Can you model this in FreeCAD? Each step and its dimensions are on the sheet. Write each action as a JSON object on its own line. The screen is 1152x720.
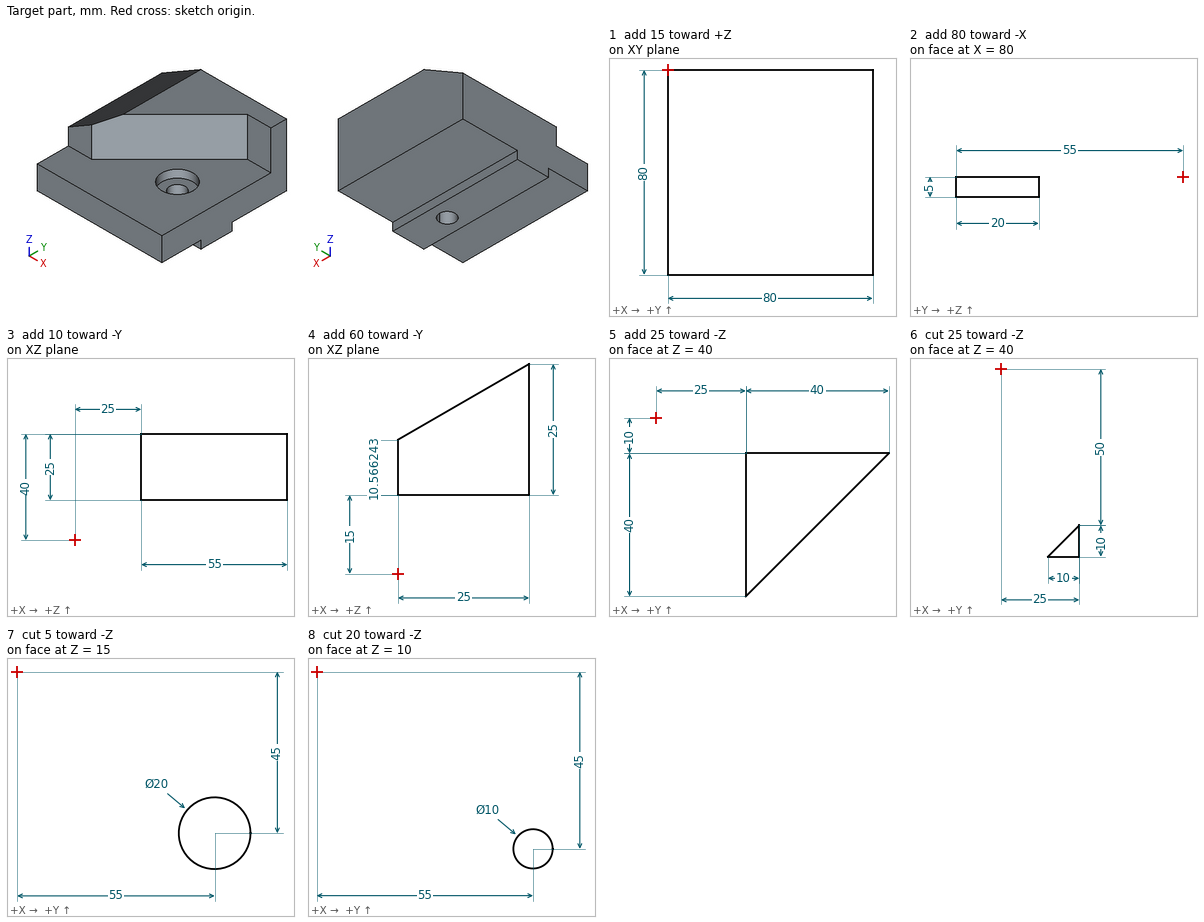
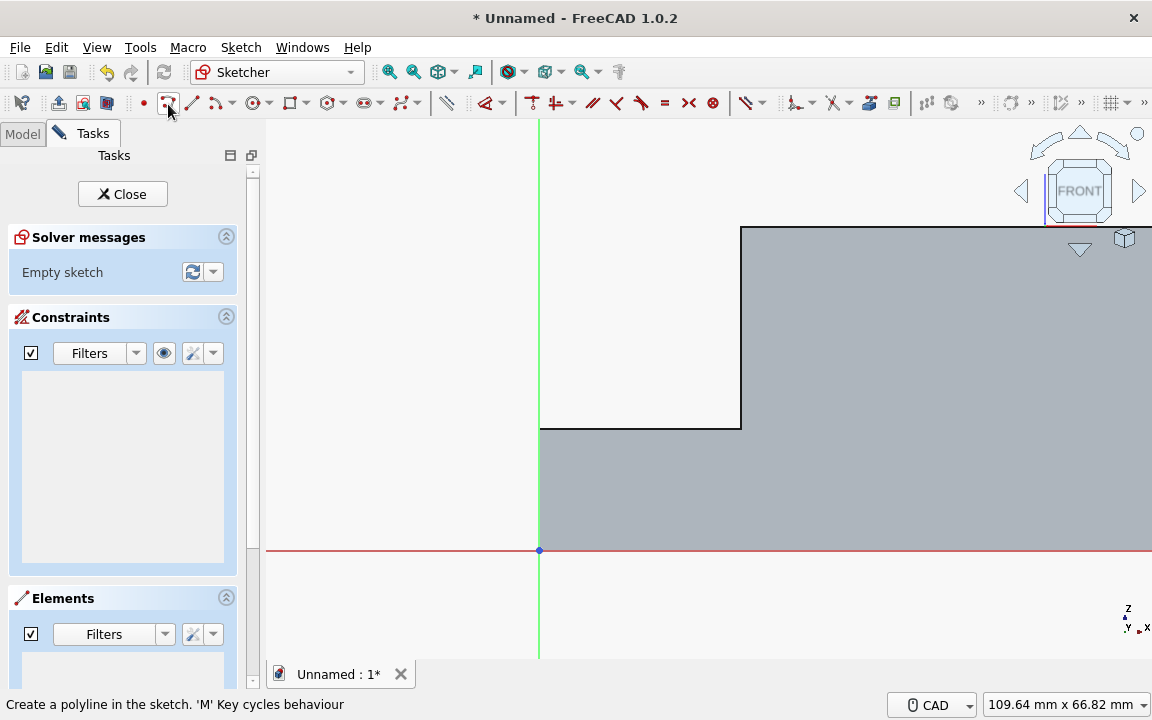
{"action": "left_click", "coordinate": [539, 429]}
{"action": "left_click", "coordinate": [548, 344]}
{"action": "left_click", "coordinate": [741, 227]}
{"action": "left_click", "coordinate": [741, 429]}
{"action": "left_click", "coordinate": [539, 430]}
{"action": "key", "text": "Escape"}
{"action": "key", "text": "Escape"}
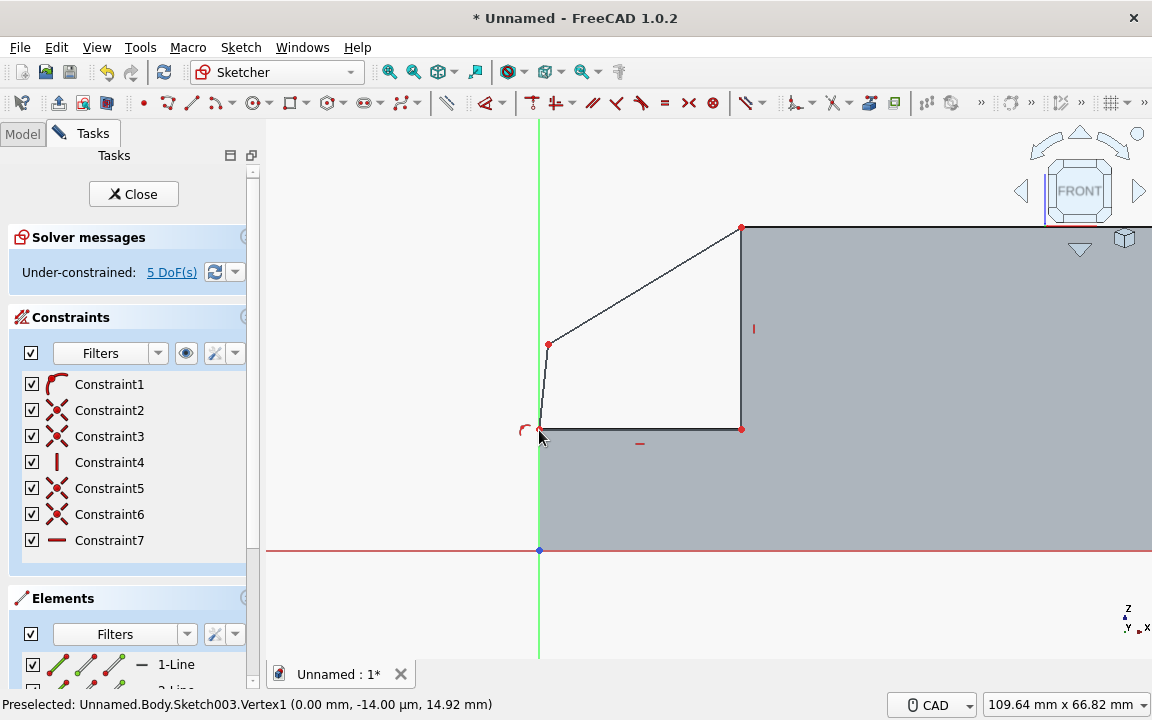
{"action": "left_click", "coordinate": [542, 404]}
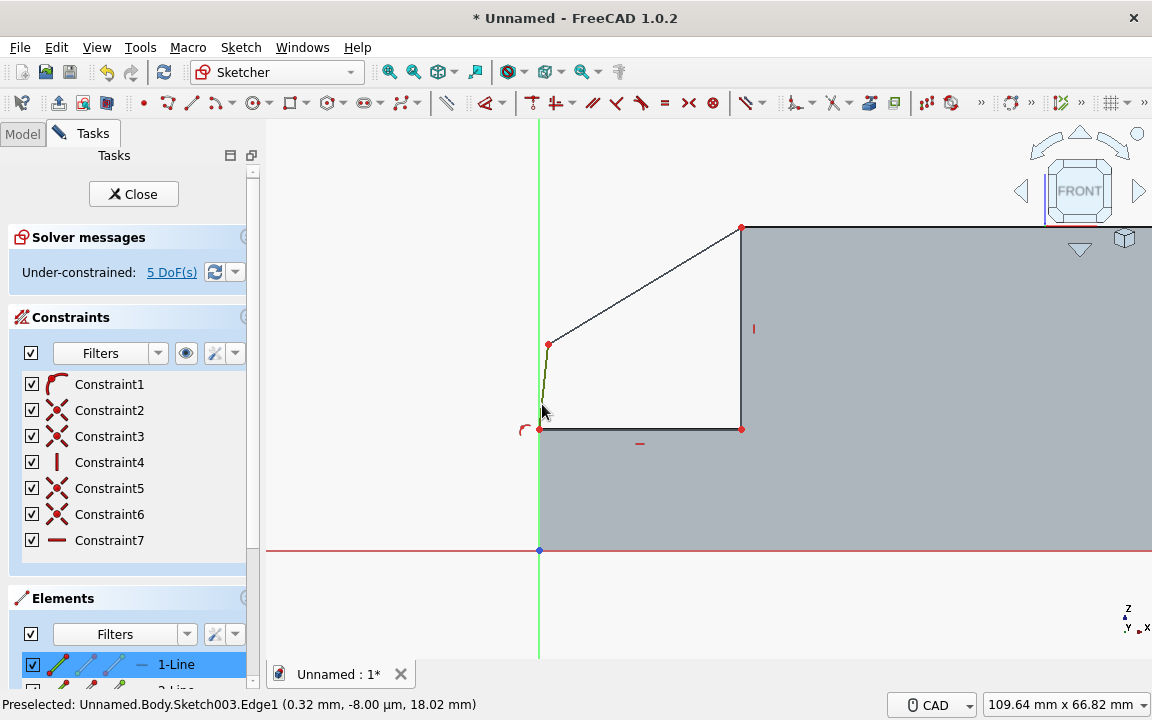
{"action": "left_click", "coordinate": [574, 104]}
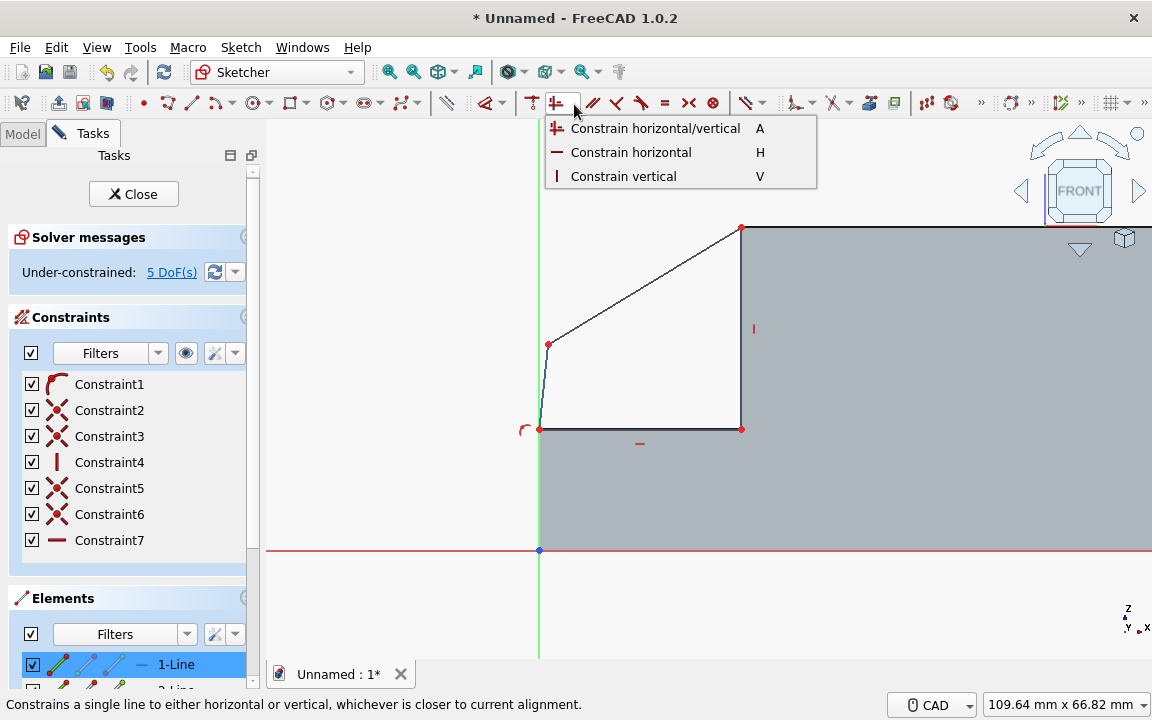
{"action": "left_click", "coordinate": [681, 176]}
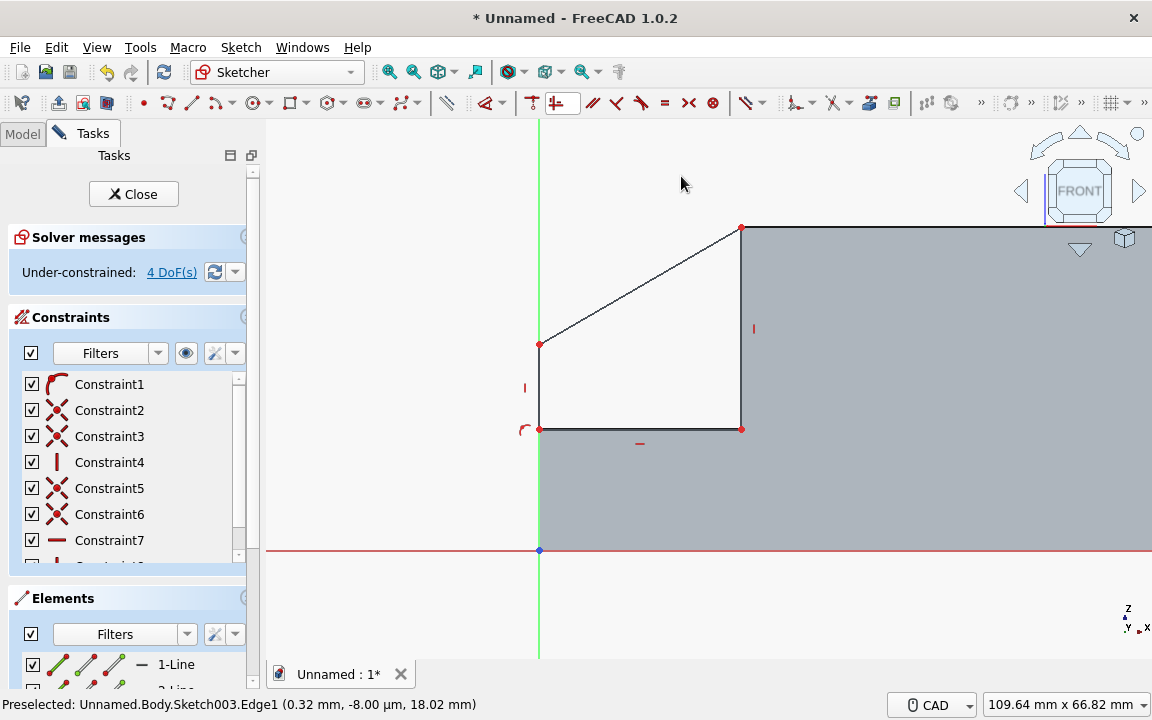
{"action": "left_click", "coordinate": [486, 104]}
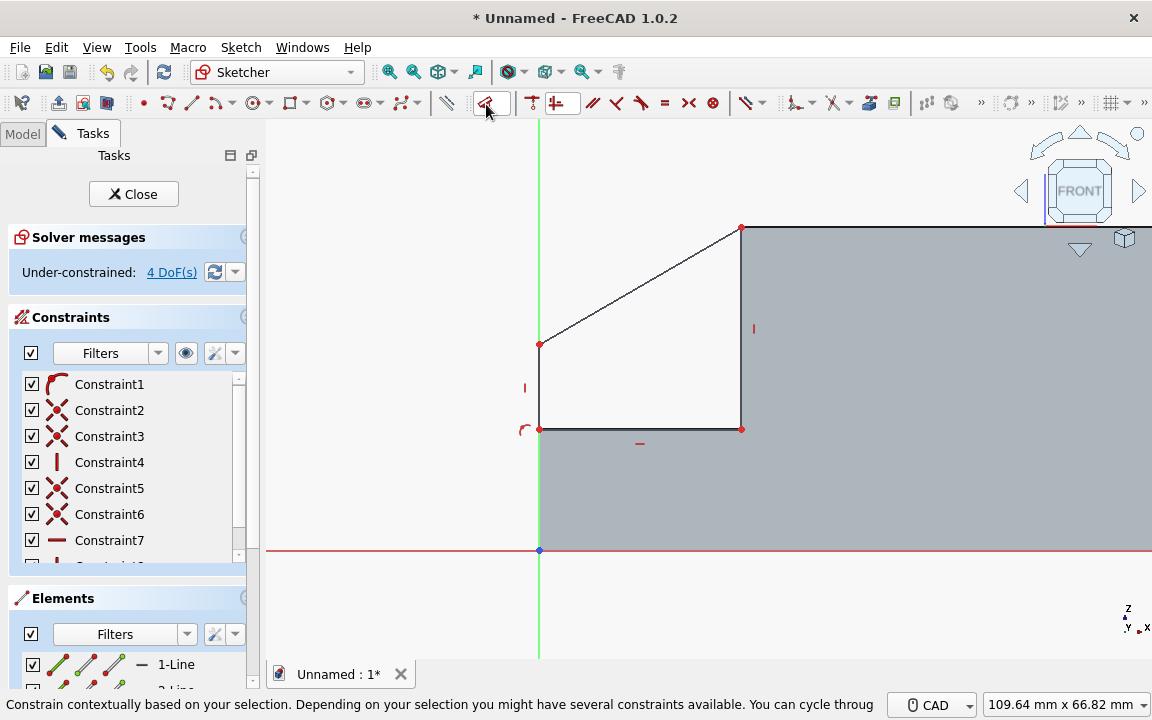
{"action": "left_click", "coordinate": [741, 289]}
{"action": "left_click", "coordinate": [775, 329]}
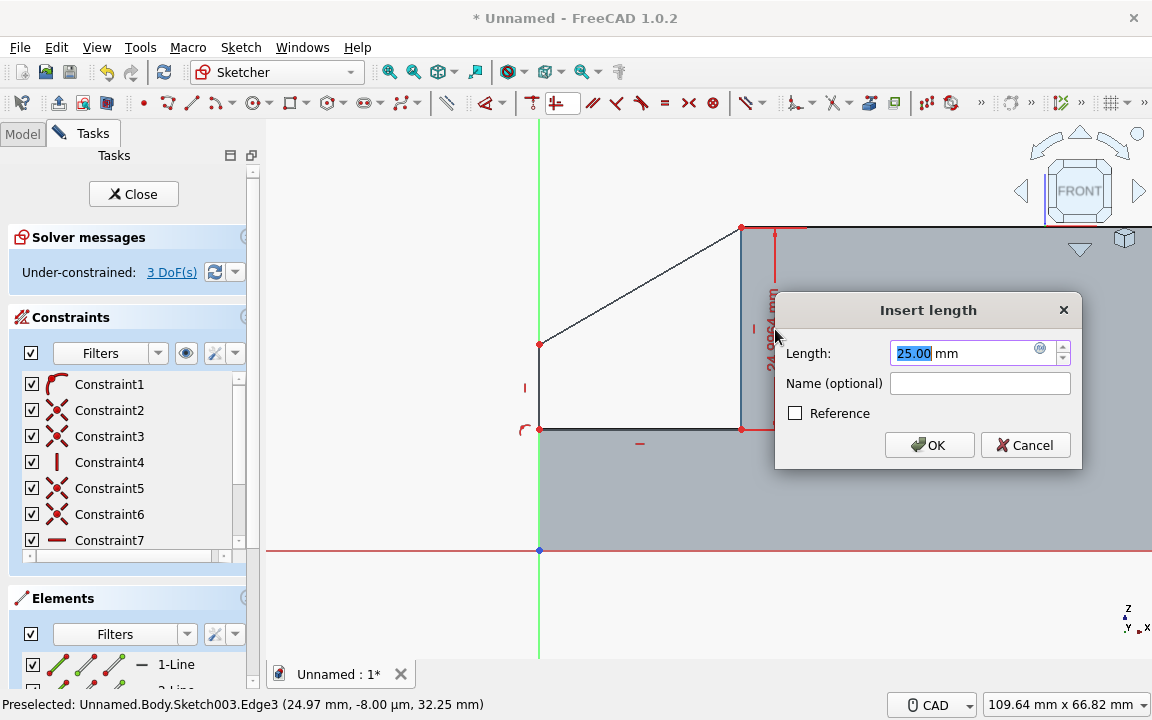
{"action": "type", "text": "25"}
{"action": "key", "text": "Return"}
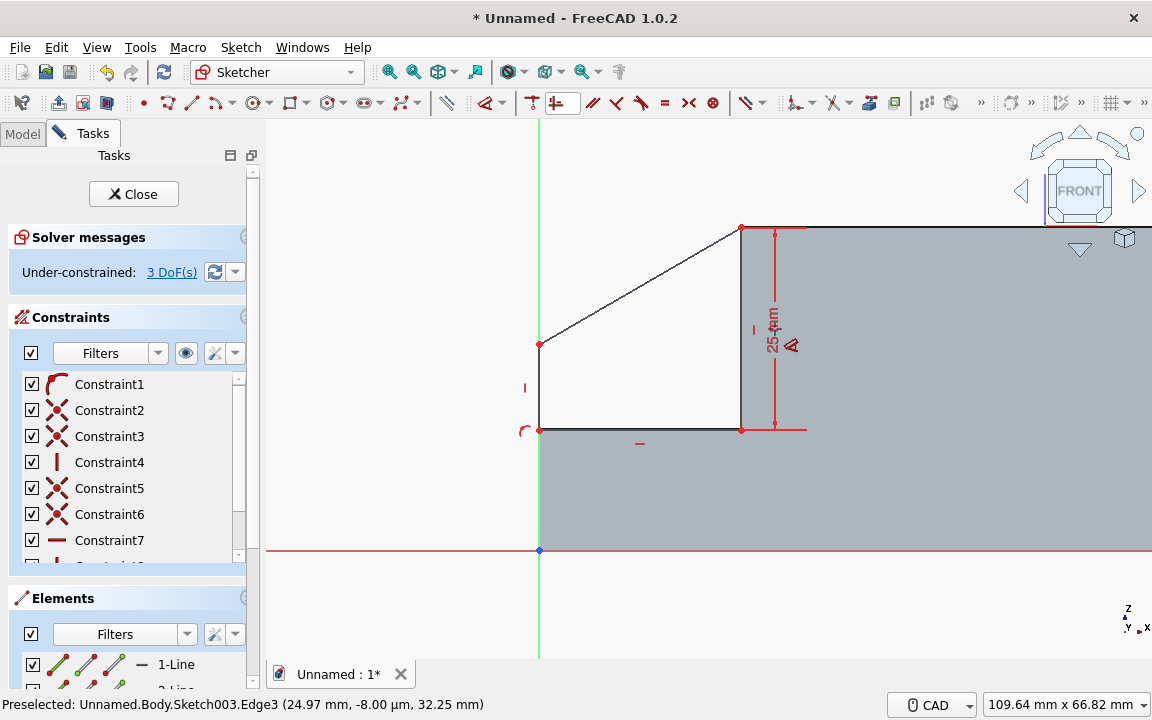
{"action": "left_click", "coordinate": [680, 430]}
{"action": "left_click", "coordinate": [640, 464]}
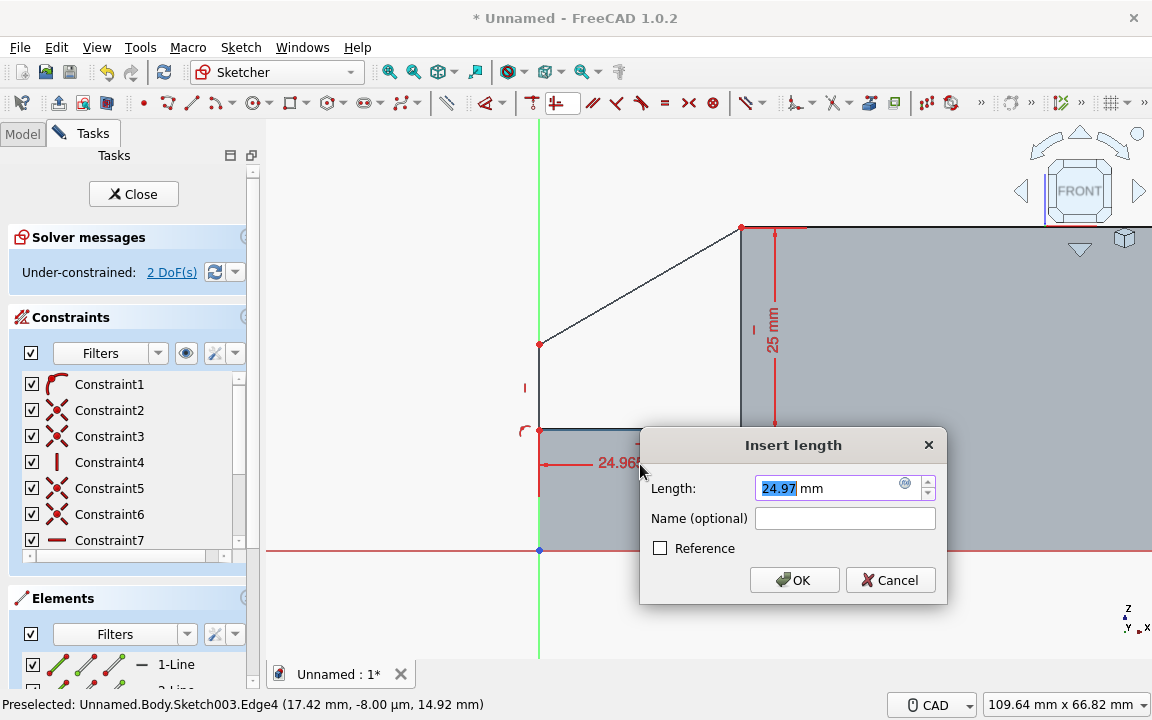
{"action": "type", "text": "25"}
{"action": "key", "text": "Return"}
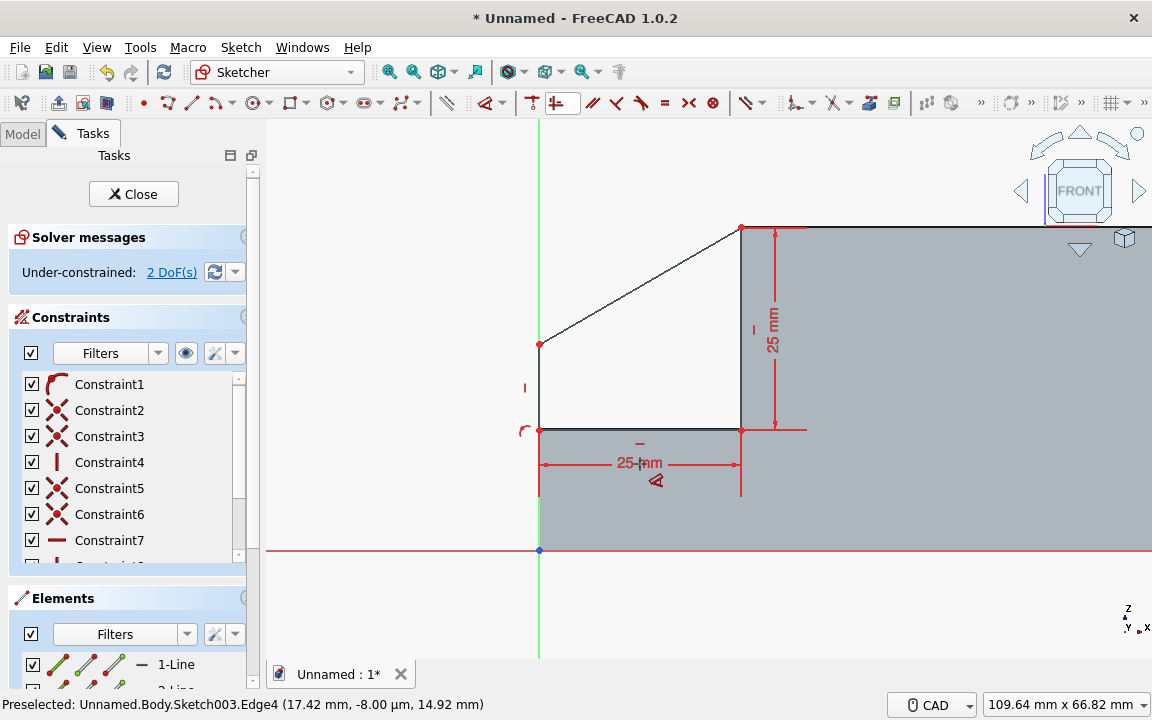
{"action": "left_click", "coordinate": [539, 430]}
{"action": "left_click", "coordinate": [505, 490]}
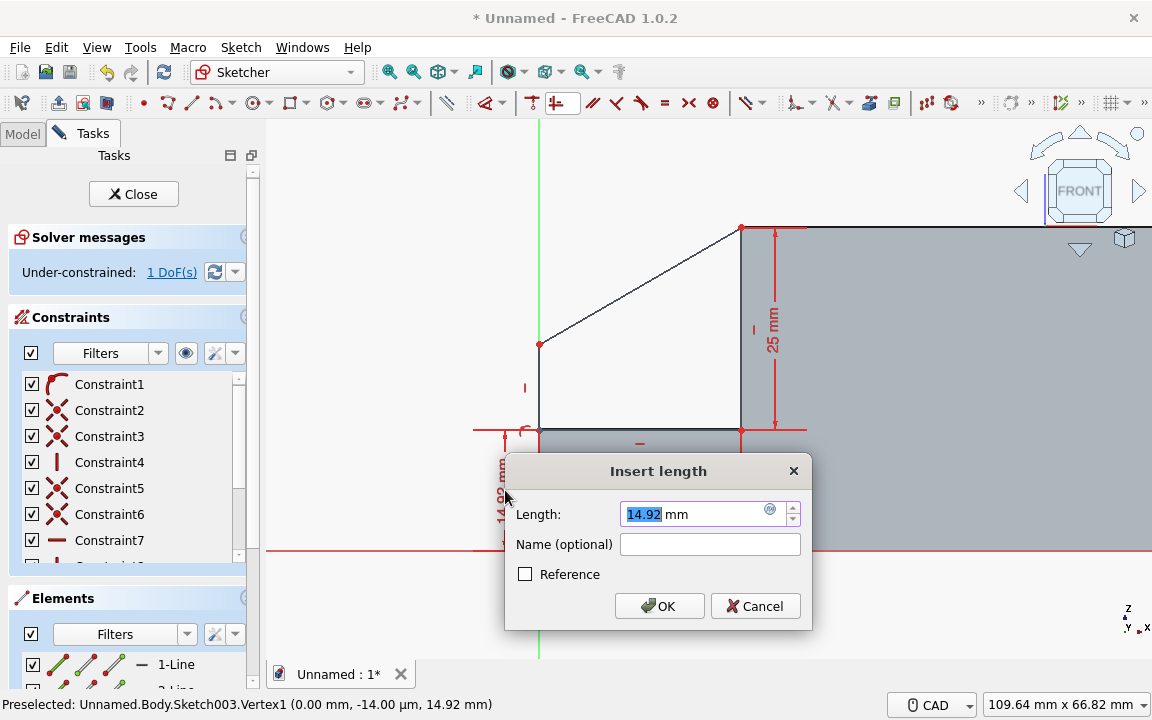
{"action": "type", "text": "15"}
{"action": "key", "text": "Return"}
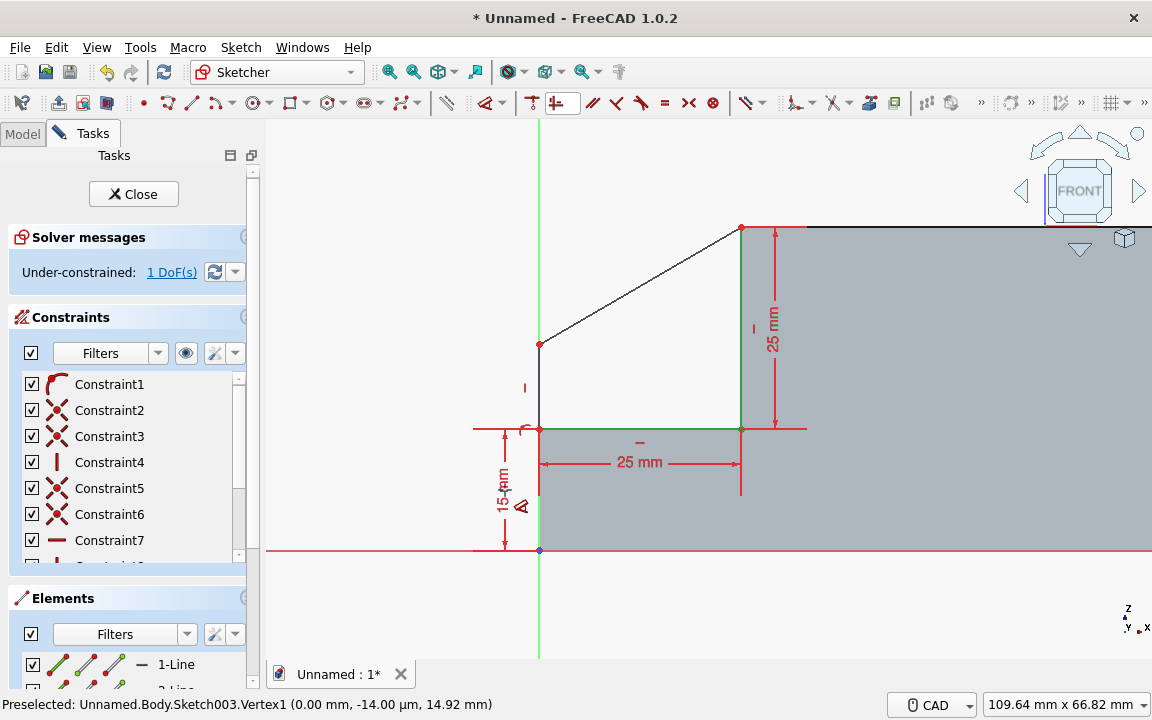
{"action": "left_click", "coordinate": [539, 404]}
{"action": "left_click", "coordinate": [505, 387]}